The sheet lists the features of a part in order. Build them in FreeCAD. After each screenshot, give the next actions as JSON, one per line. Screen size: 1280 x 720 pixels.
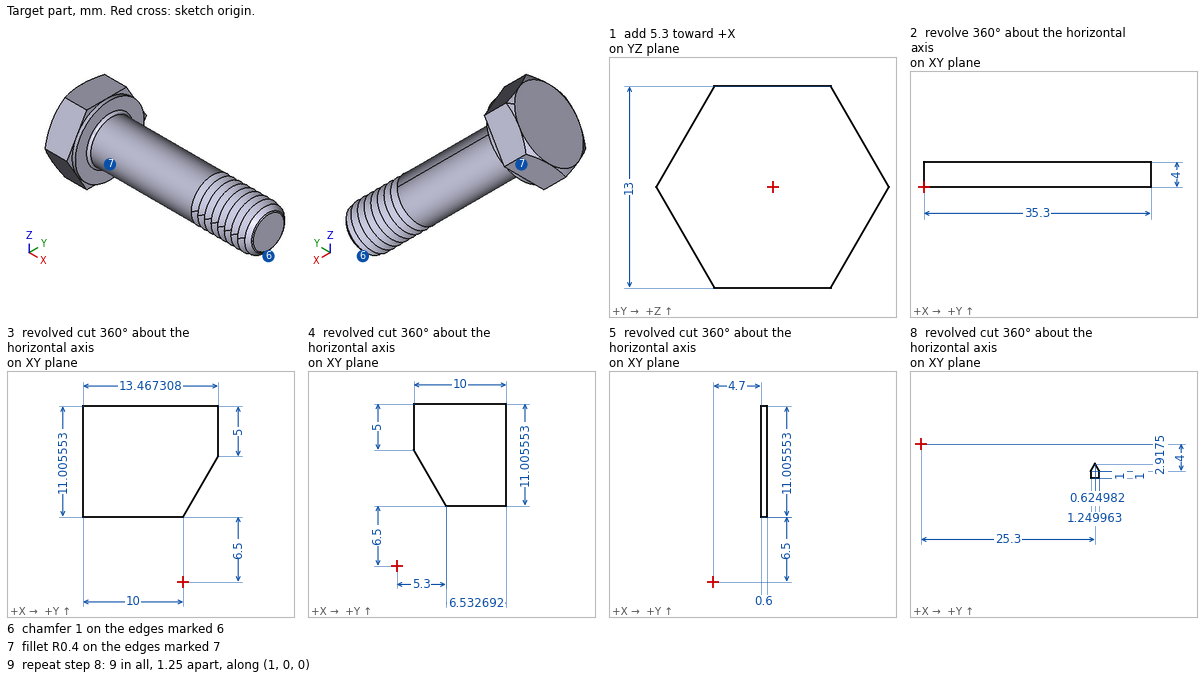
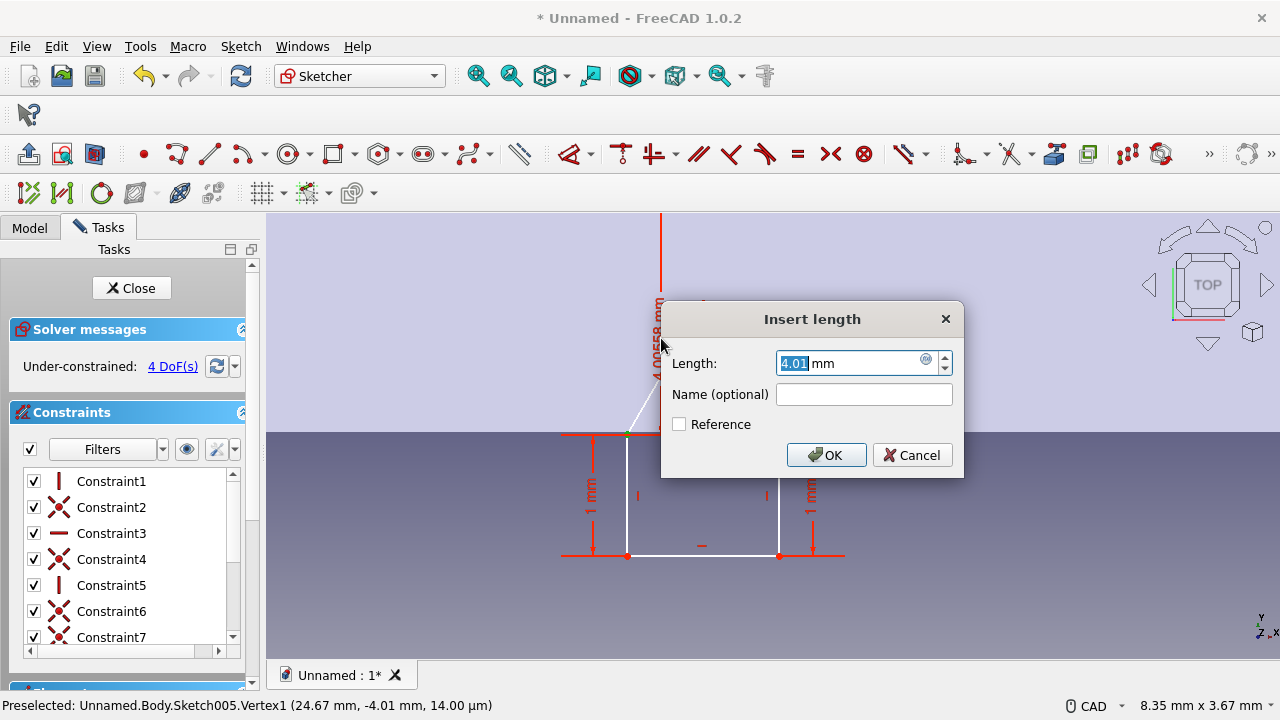
{"action": "type", "text": "4"}
{"action": "key", "text": "Return"}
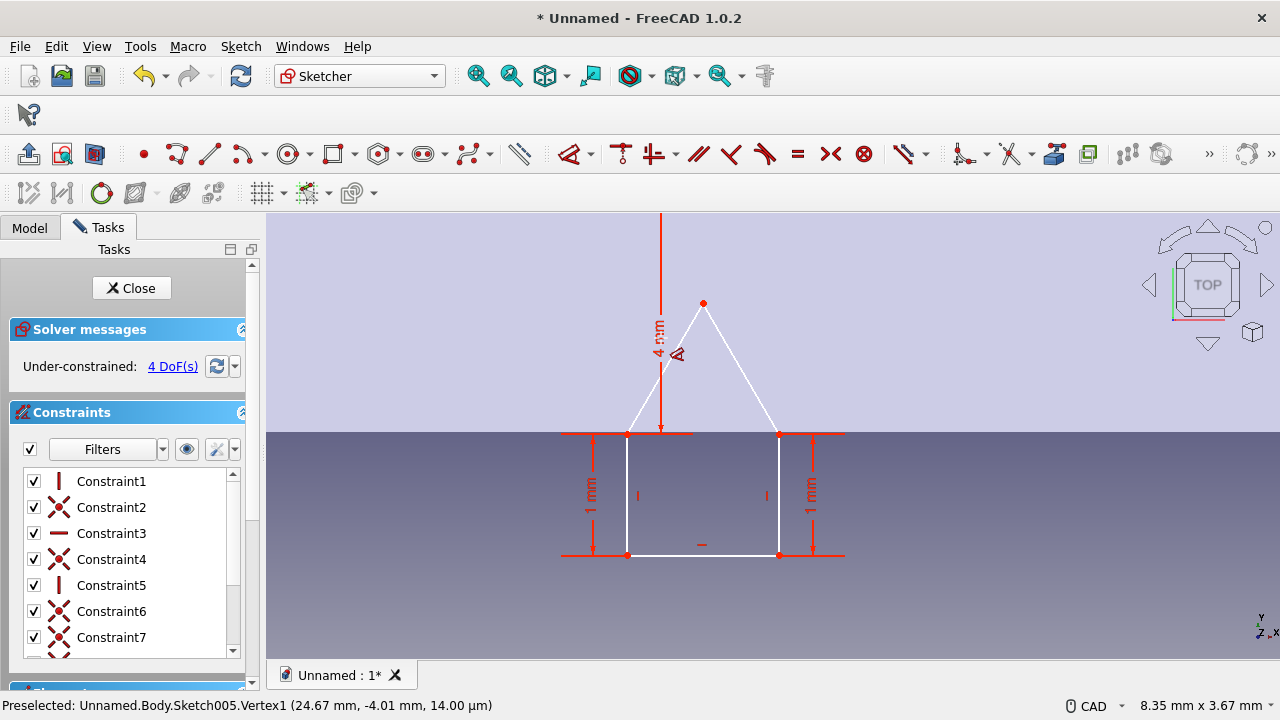
{"action": "left_click", "coordinate": [703, 304]}
{"action": "left_click", "coordinate": [499, 338]}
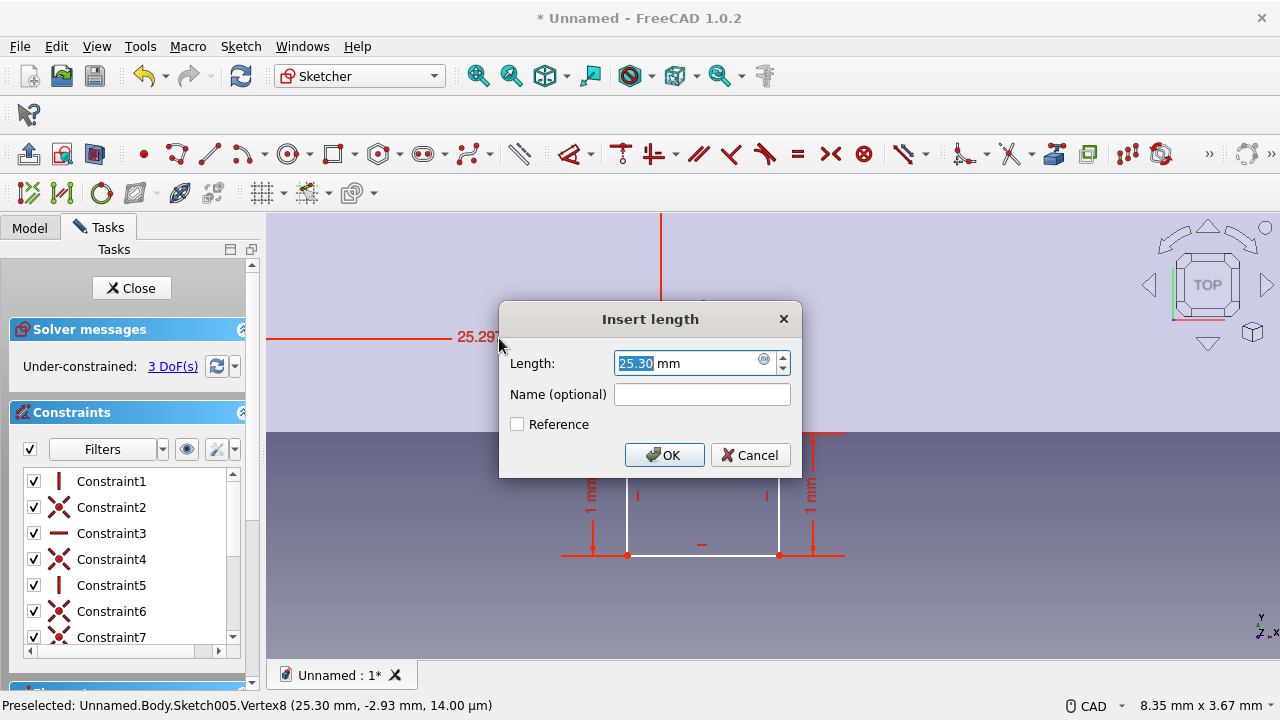
{"action": "type", "text": "25.3"}
{"action": "key", "text": "Return"}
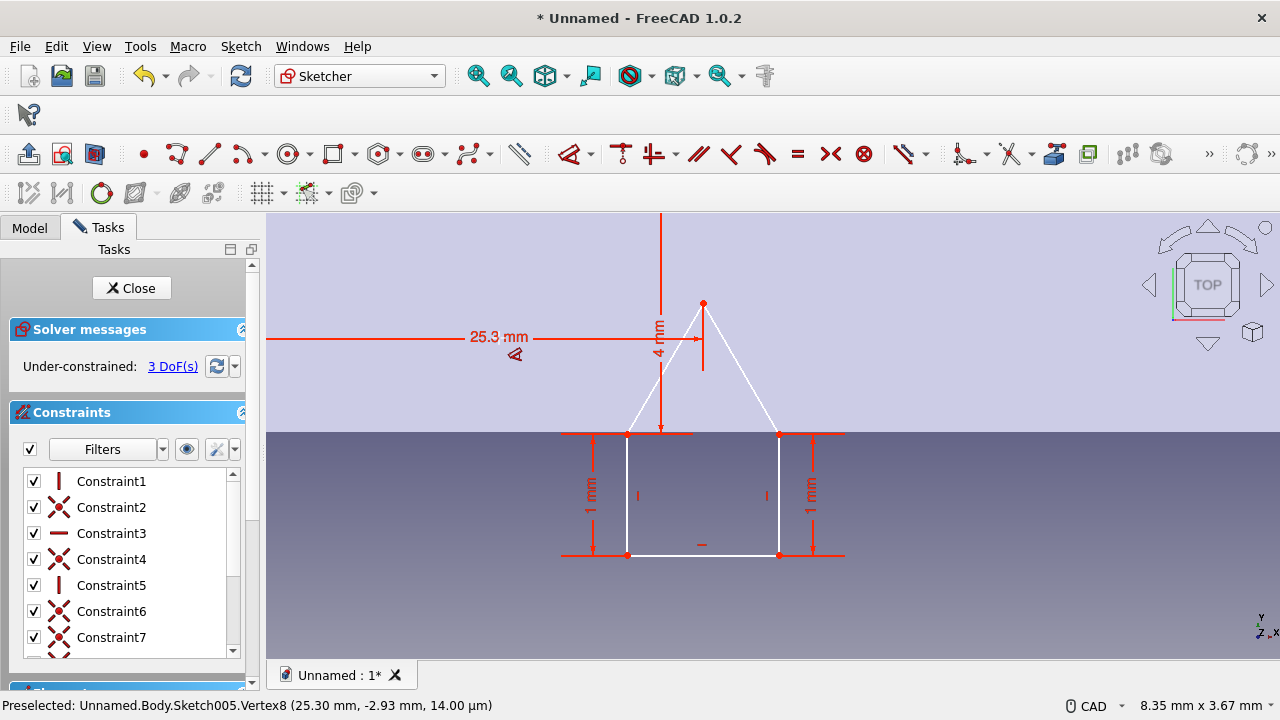
{"action": "left_click", "coordinate": [703, 304]}
{"action": "left_click", "coordinate": [737, 273]}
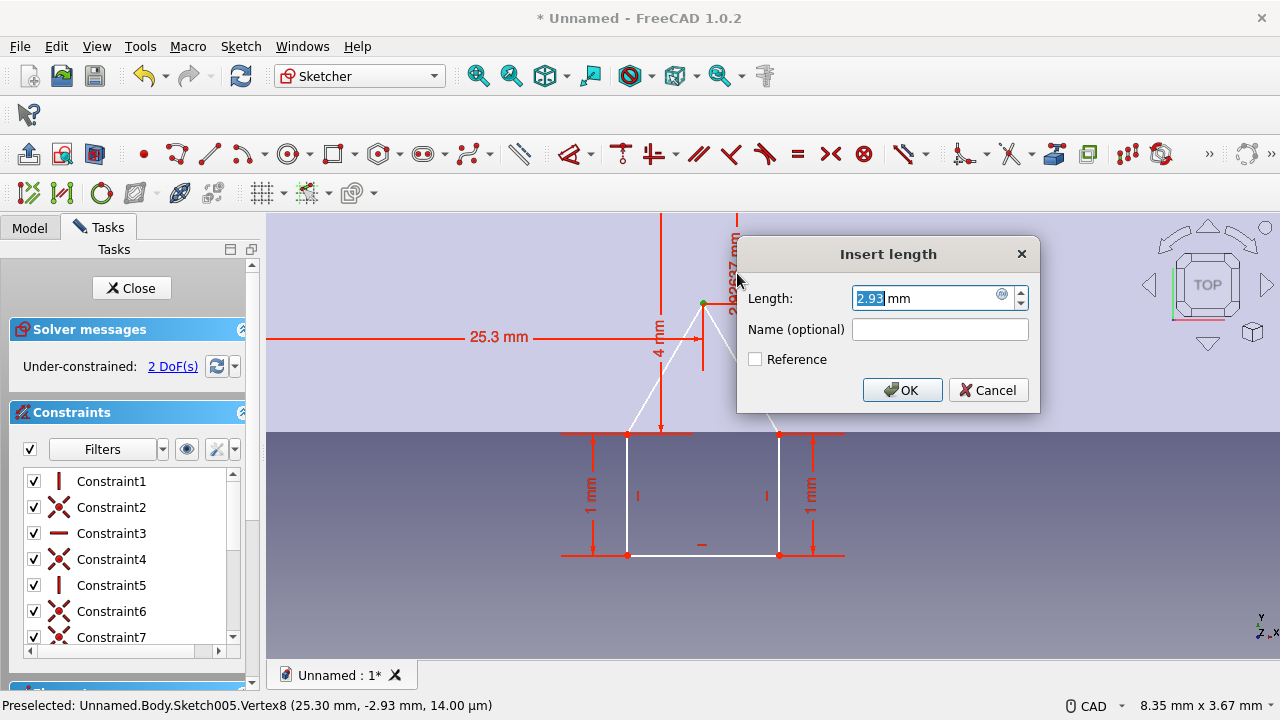
{"action": "type", "text": "2.9175"}
{"action": "key", "text": "Return"}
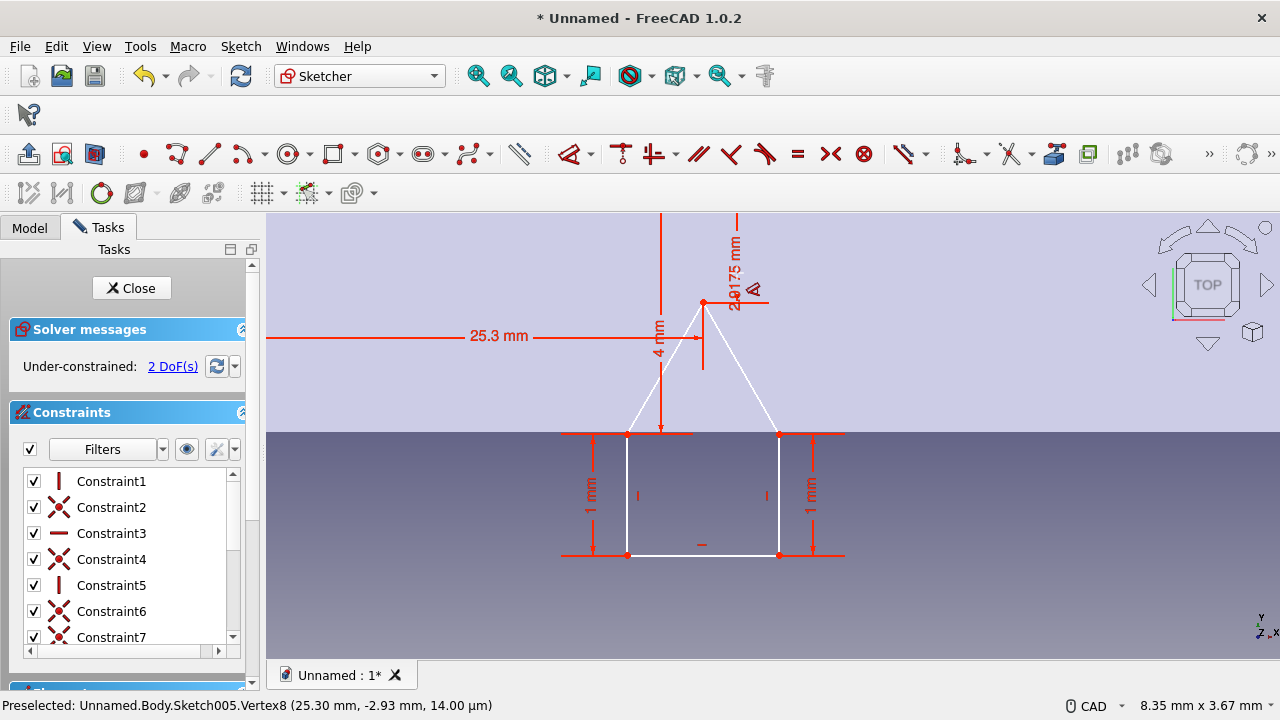
{"action": "left_click", "coordinate": [673, 556]}
{"action": "left_click", "coordinate": [703, 590]}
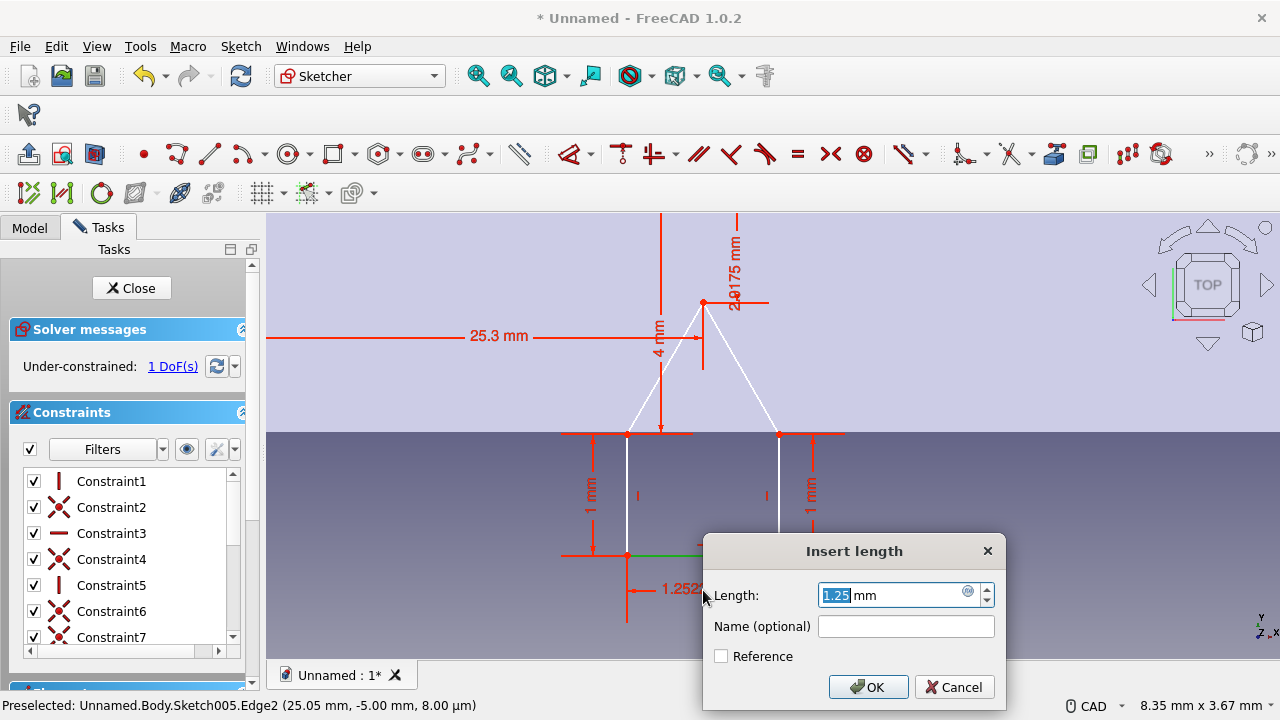
{"action": "type", "text": "1.249963"}
{"action": "key", "text": "Return"}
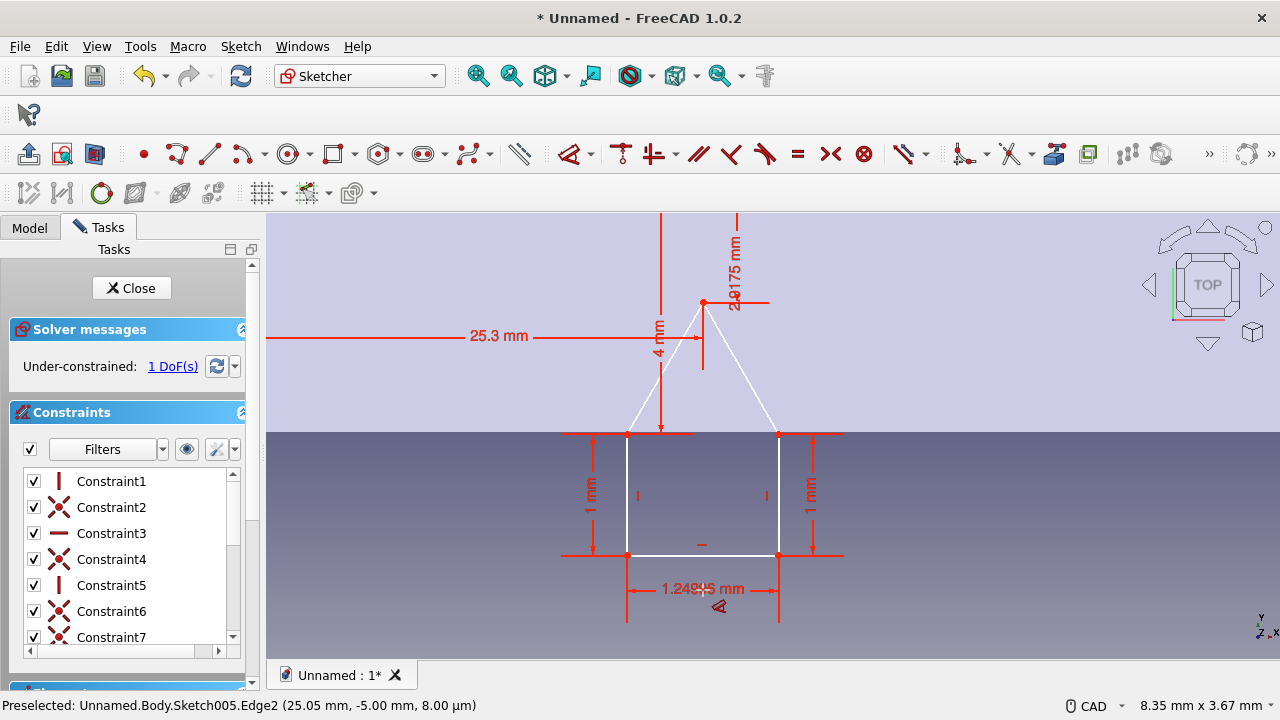
{"action": "left_click", "coordinate": [756, 395]}
{"action": "left_click", "coordinate": [741, 468]}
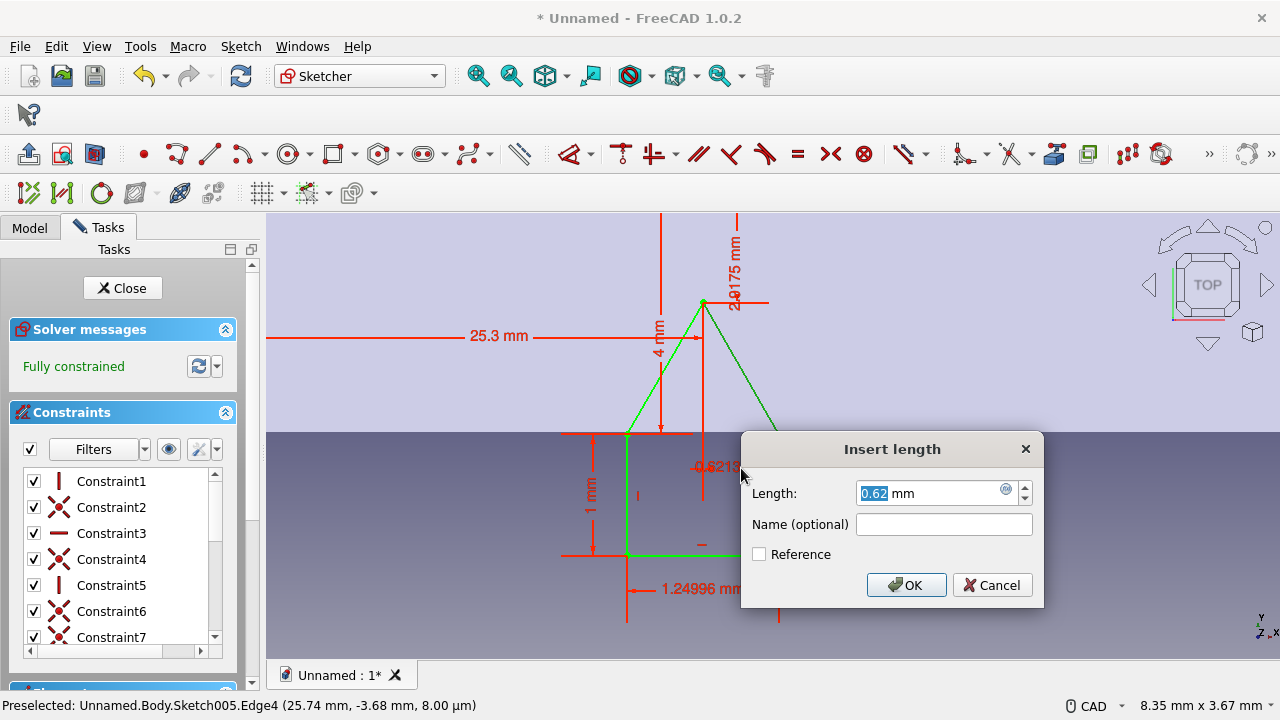
{"action": "type", "text": "0.624982"}
{"action": "key", "text": "Return"}
{"action": "key", "text": "Escape"}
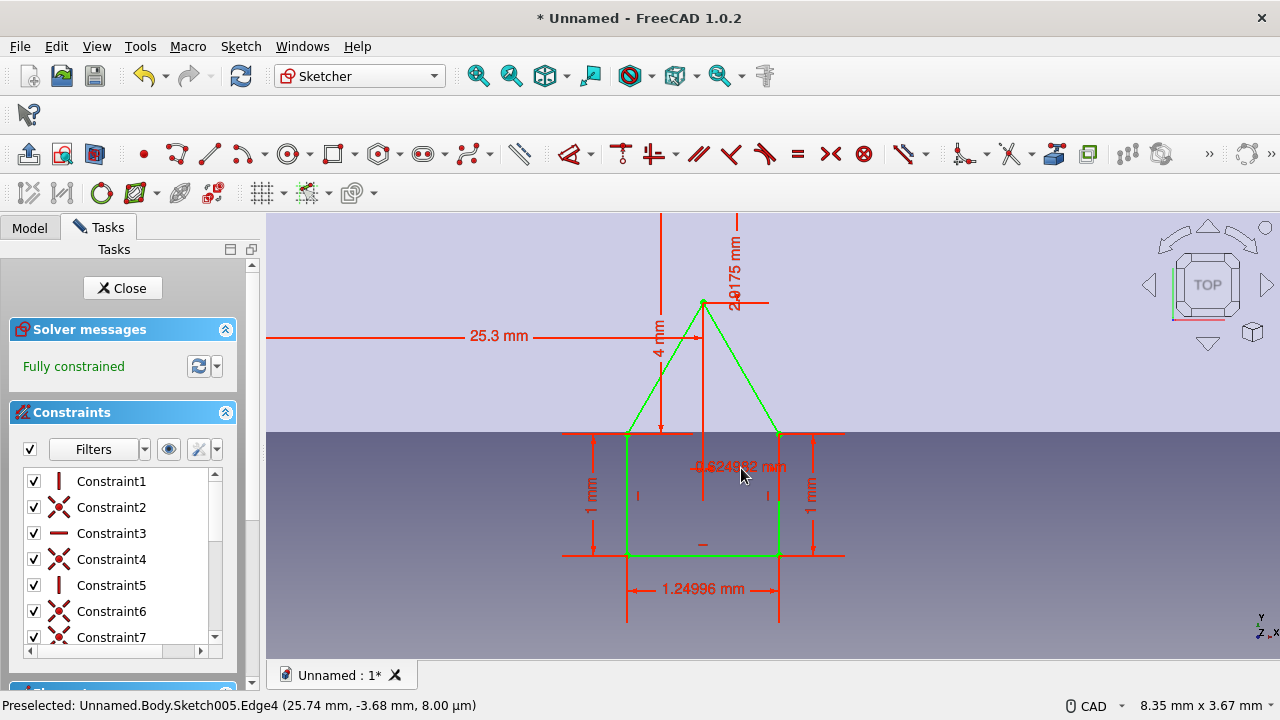
{"action": "left_click", "coordinate": [123, 288]}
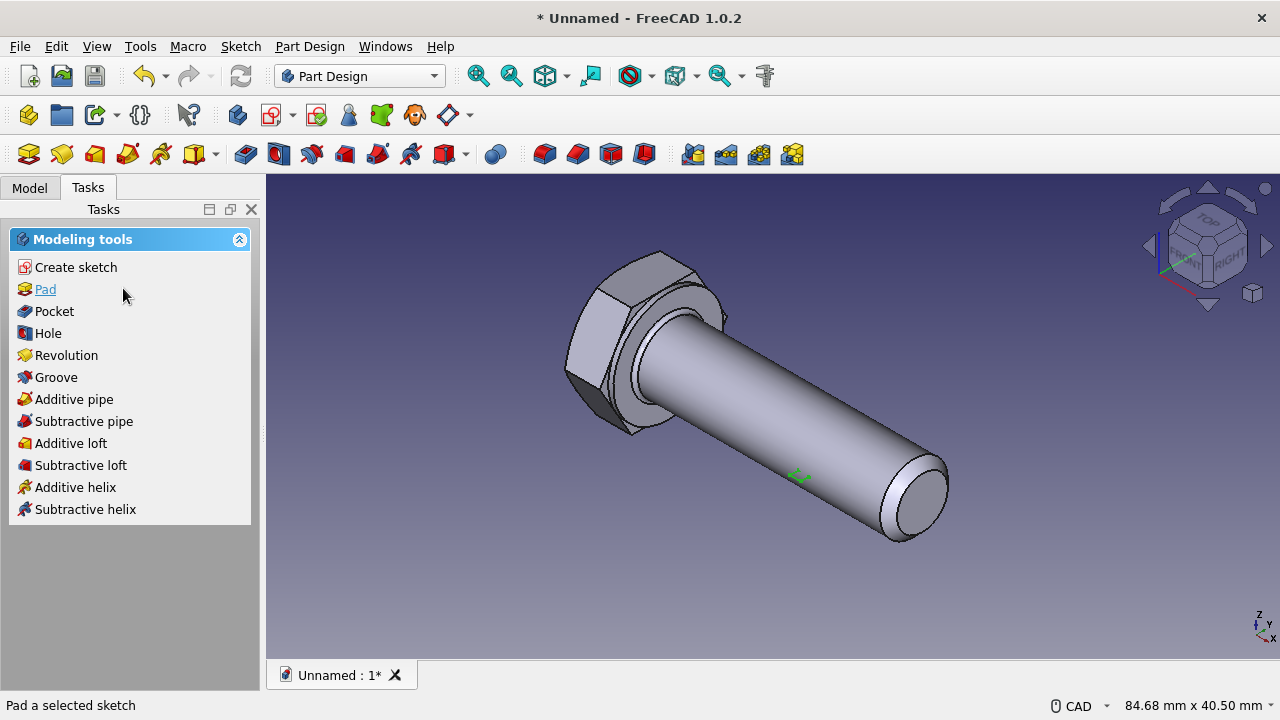
{"action": "left_click", "coordinate": [312, 154]}